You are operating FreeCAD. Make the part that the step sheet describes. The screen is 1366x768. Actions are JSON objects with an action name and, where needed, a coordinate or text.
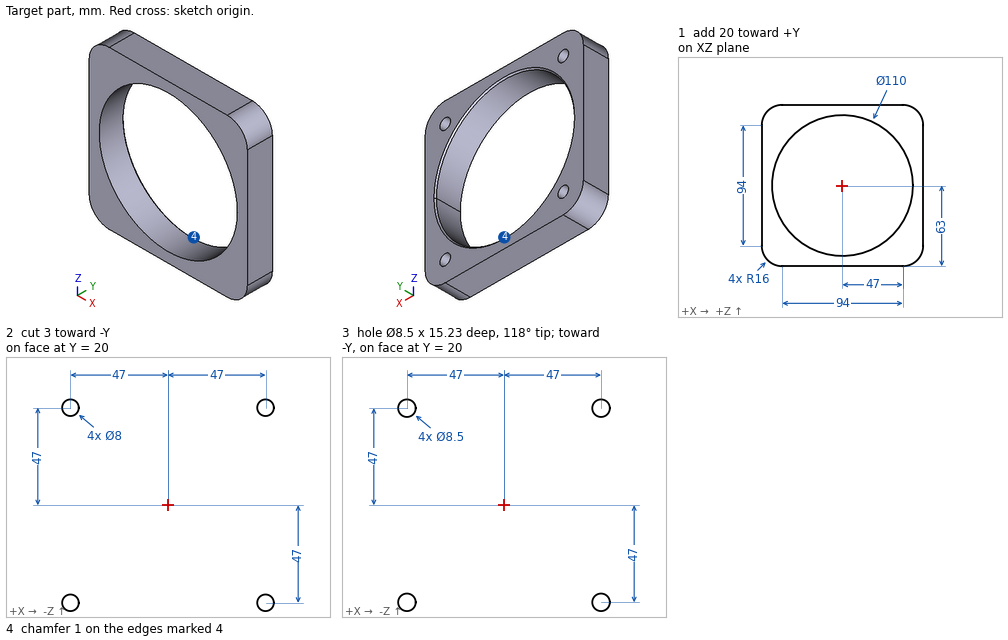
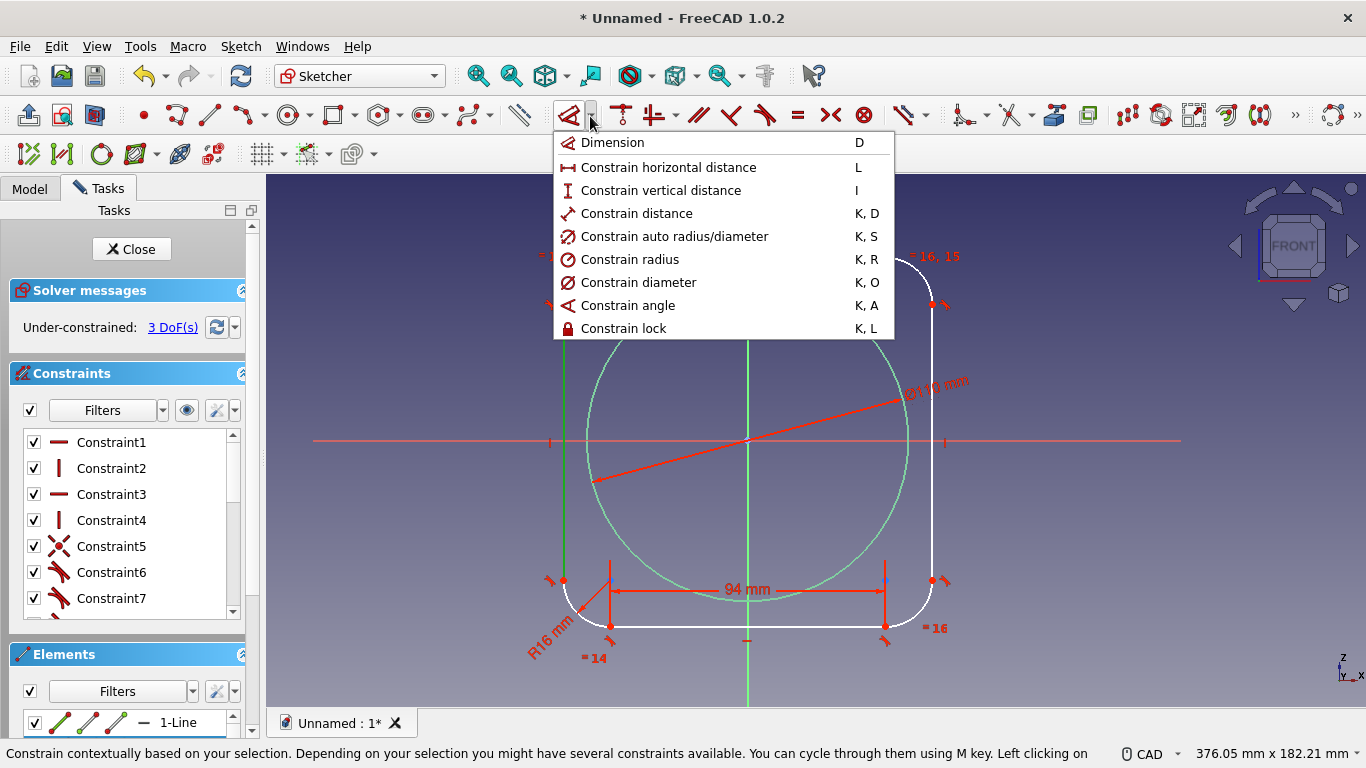
{"action": "left_click", "coordinate": [724, 190]}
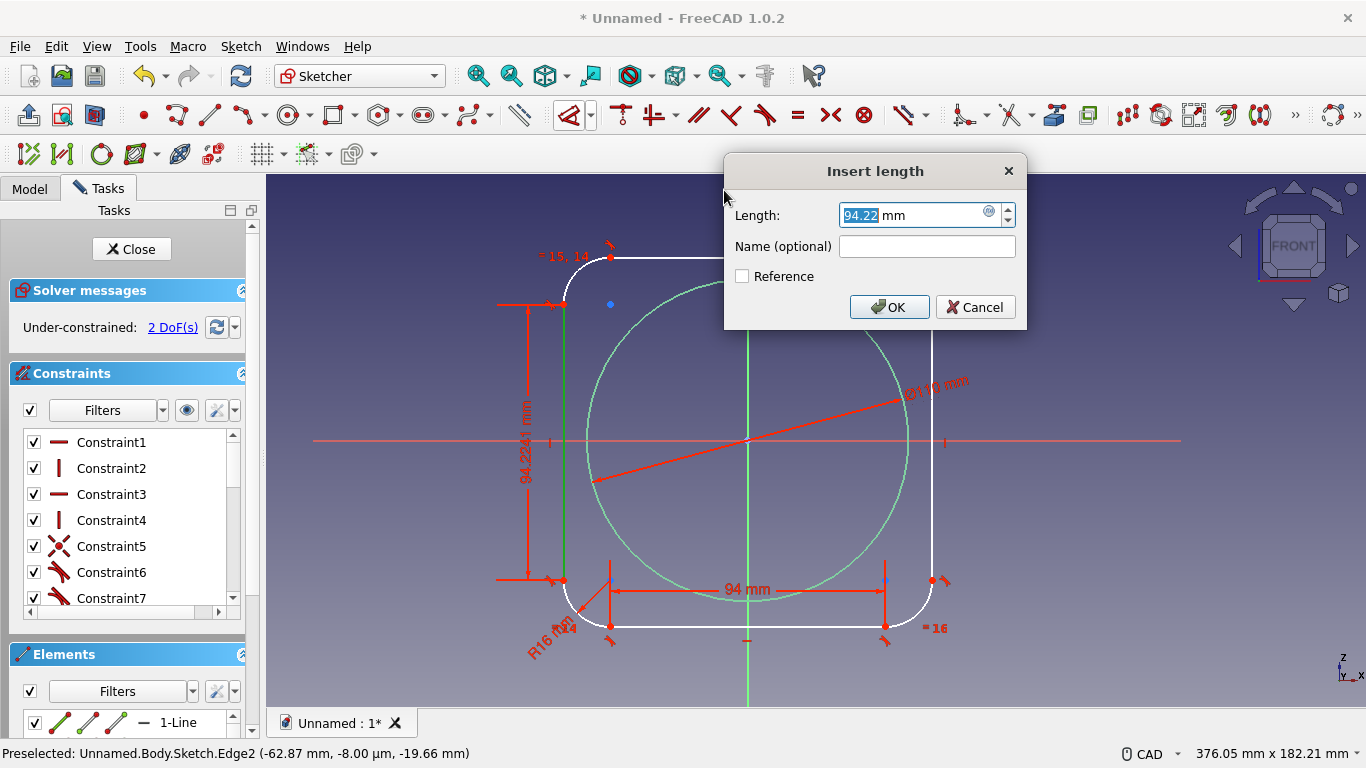
{"action": "type", "text": "94"}
{"action": "key", "text": "Return"}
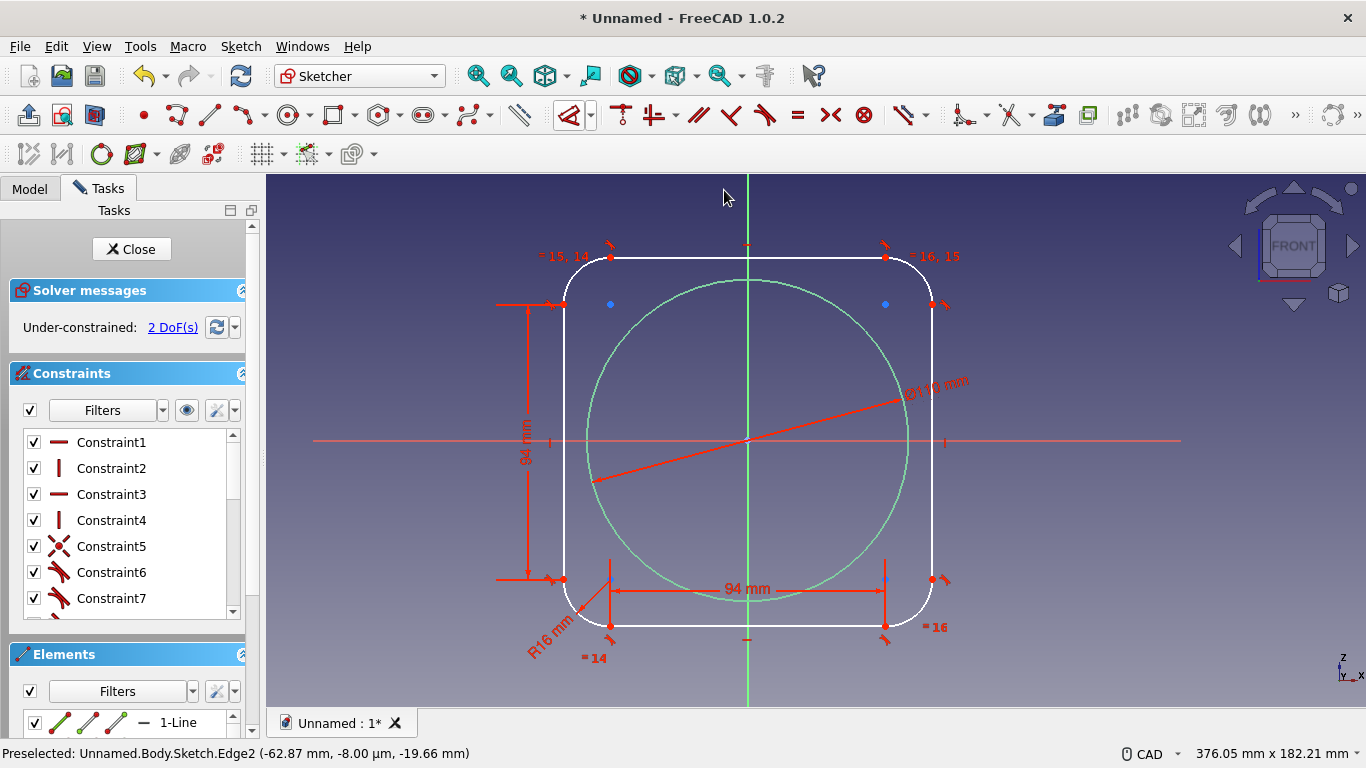
{"action": "left_click", "coordinate": [885, 626]}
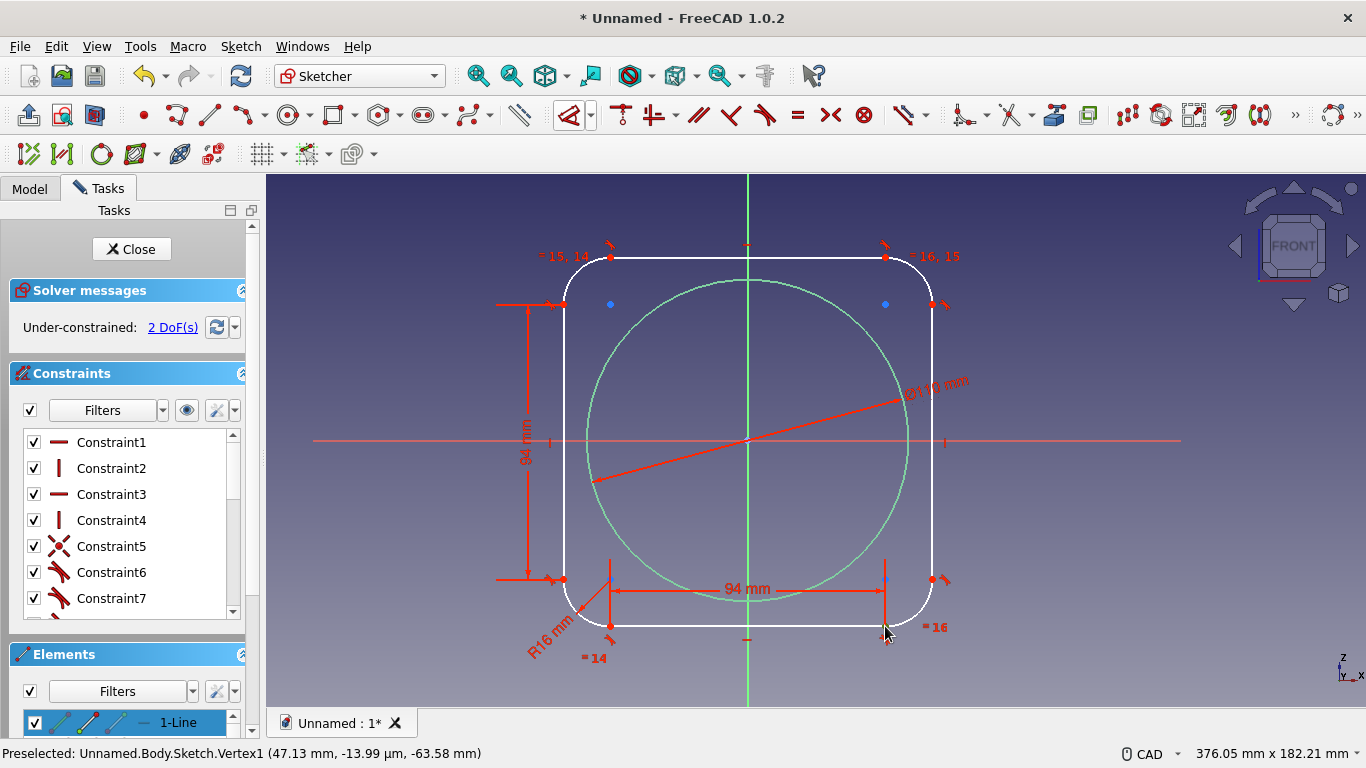
{"action": "key", "text": "l"}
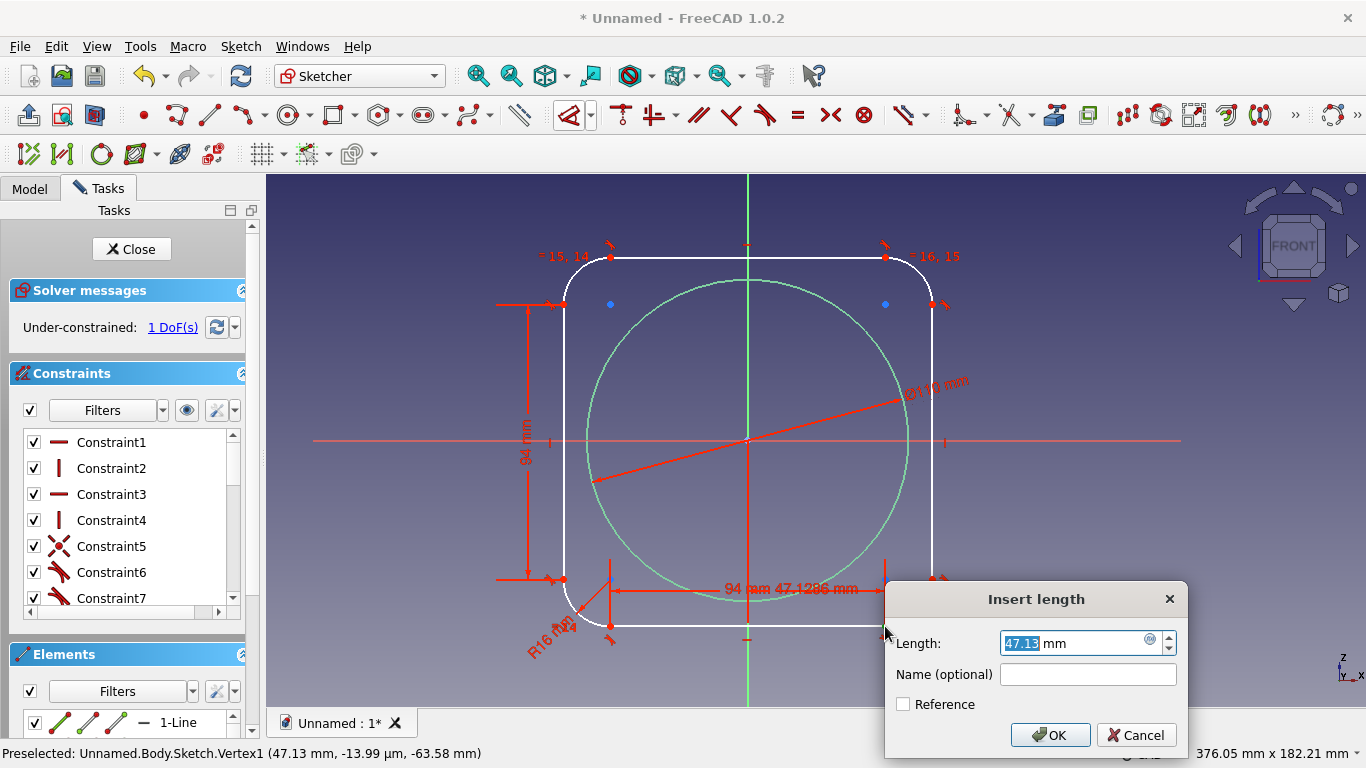
{"action": "type", "text": "47"}
{"action": "key", "text": "Return"}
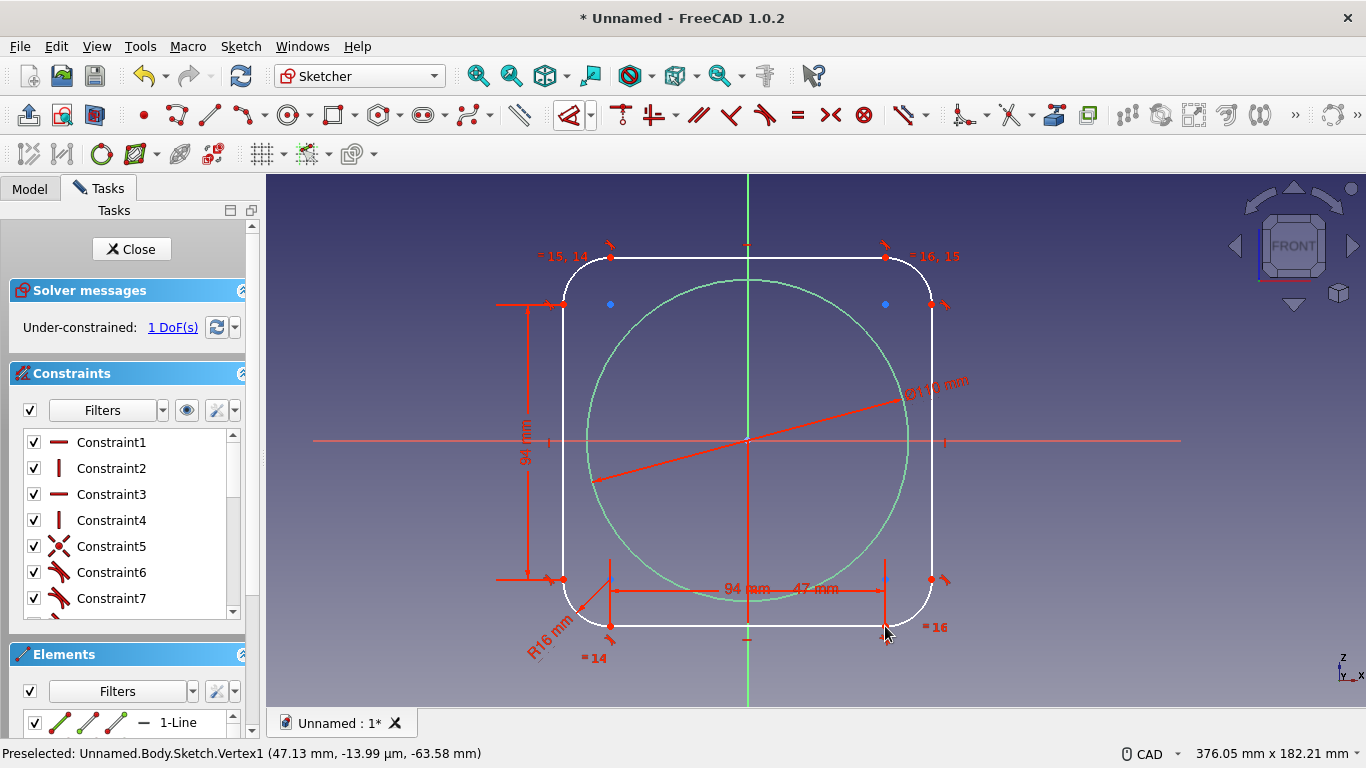
{"action": "left_click", "coordinate": [885, 626]}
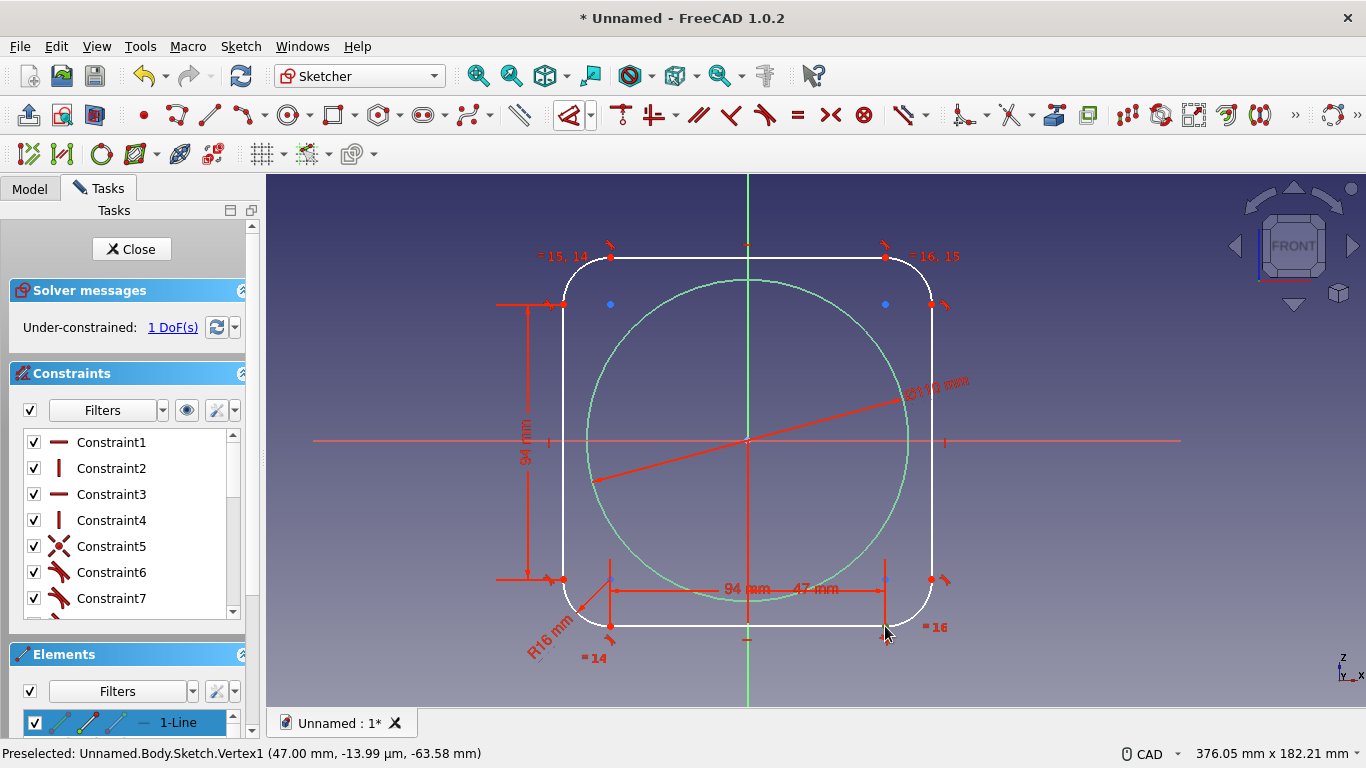
{"action": "left_click", "coordinate": [590, 116]}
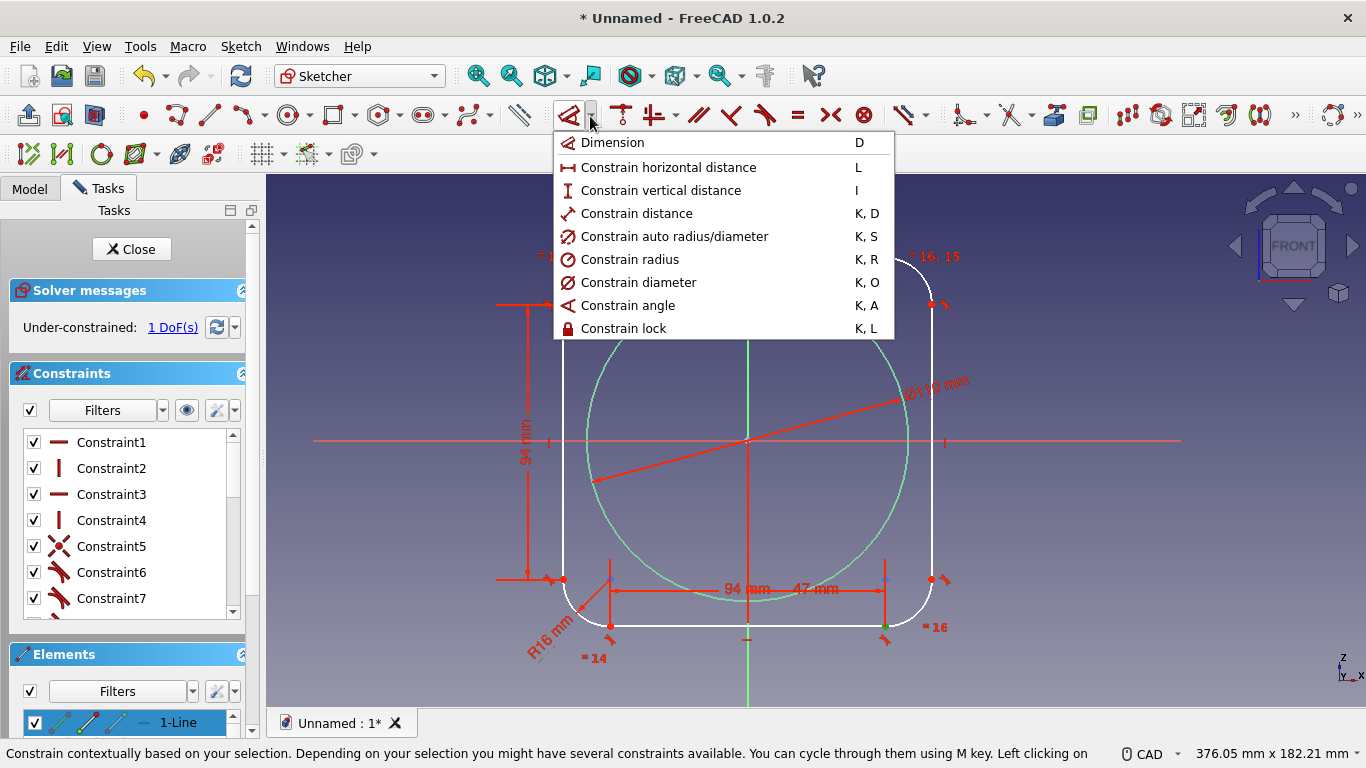
{"action": "left_click", "coordinate": [724, 190]}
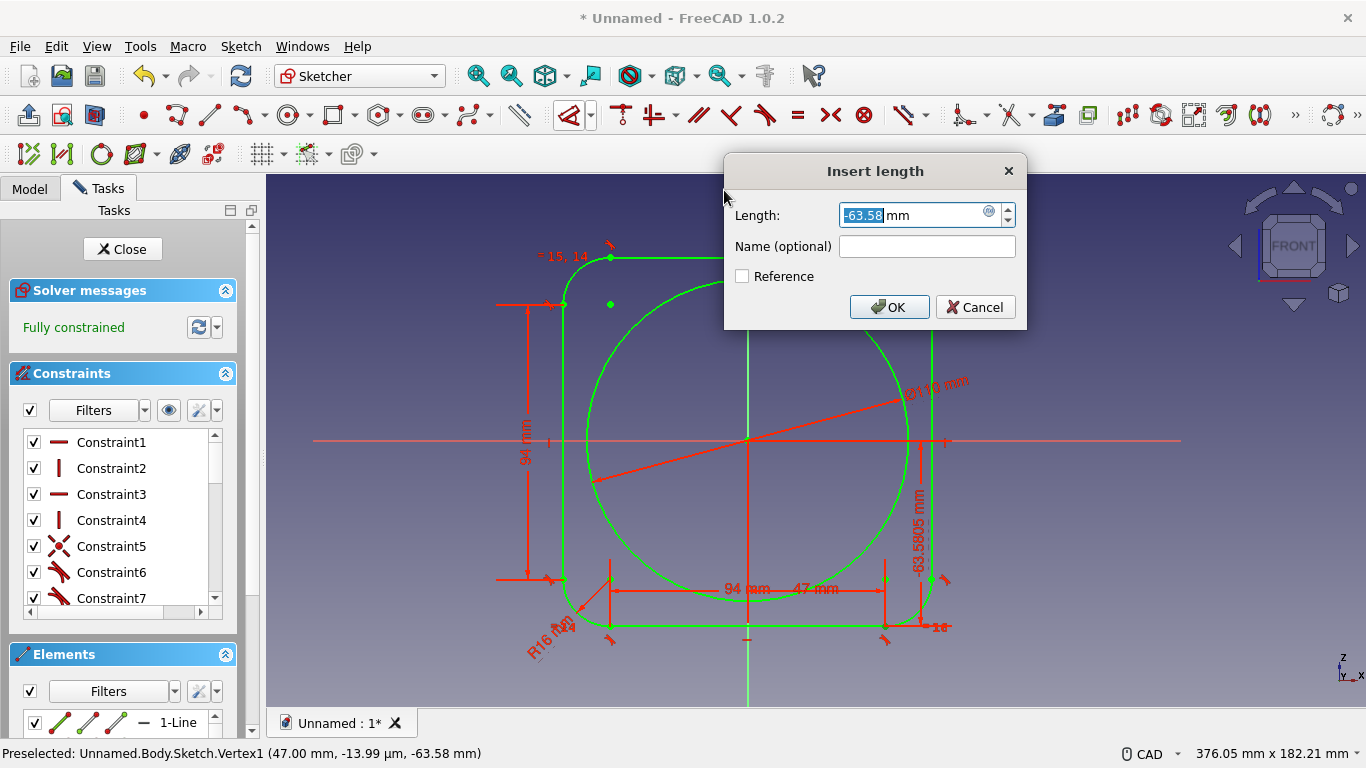
{"action": "type", "text": "-63"}
{"action": "key", "text": "Return"}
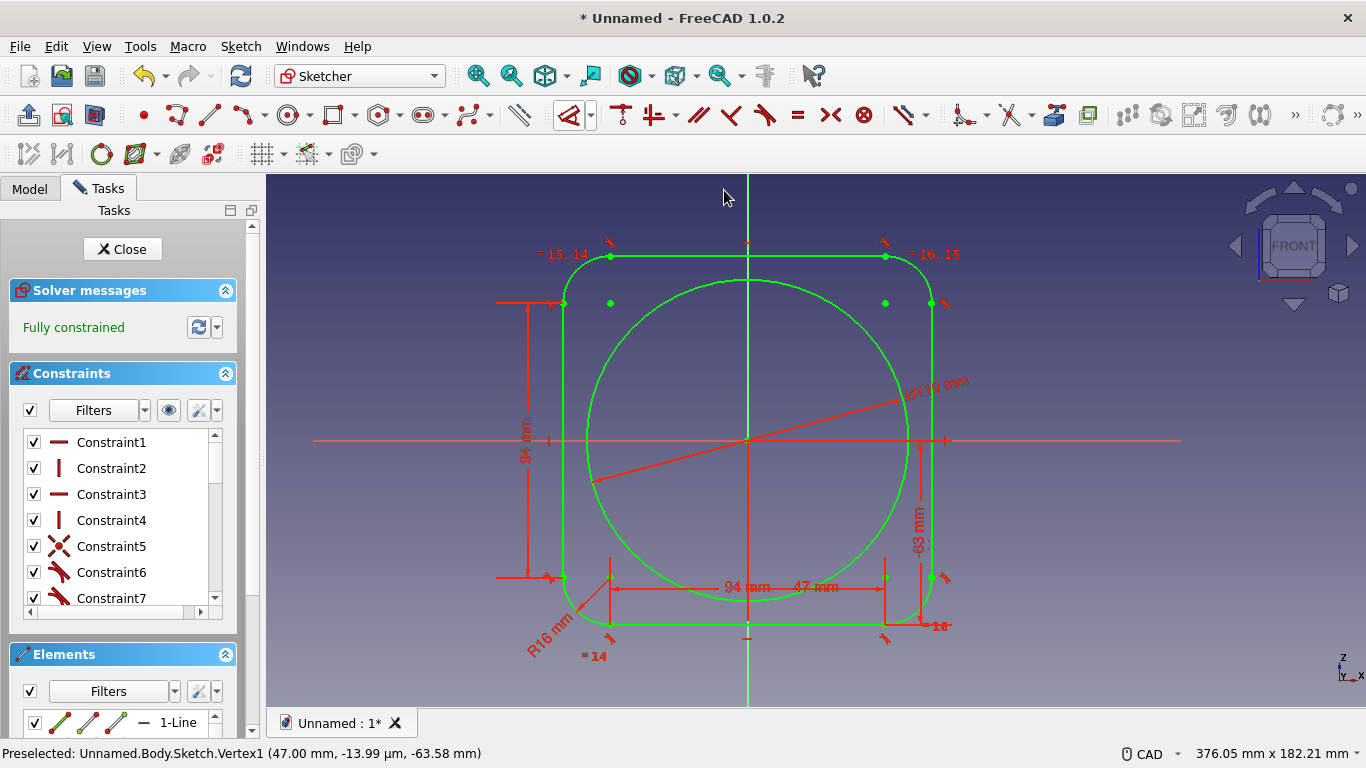
{"action": "left_click", "coordinate": [123, 249]}